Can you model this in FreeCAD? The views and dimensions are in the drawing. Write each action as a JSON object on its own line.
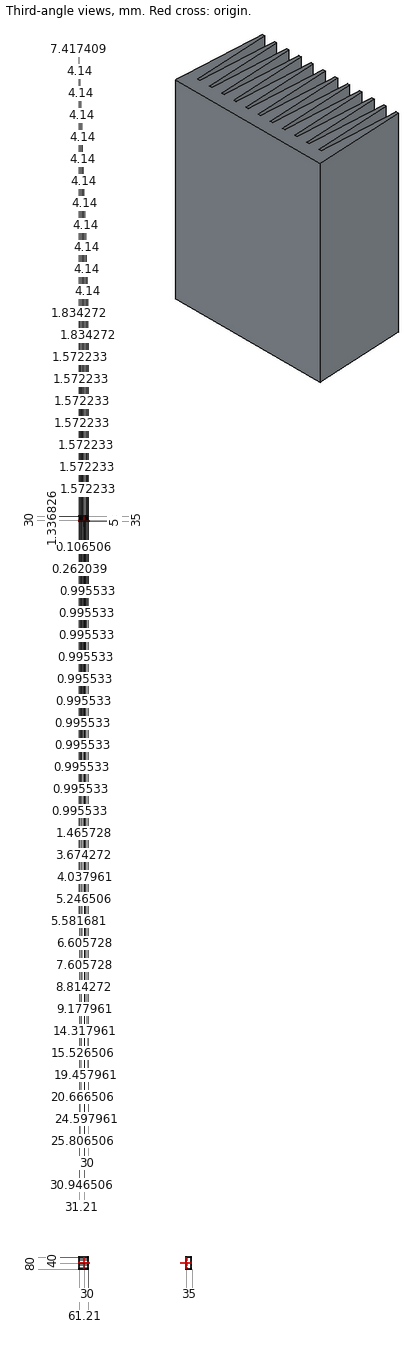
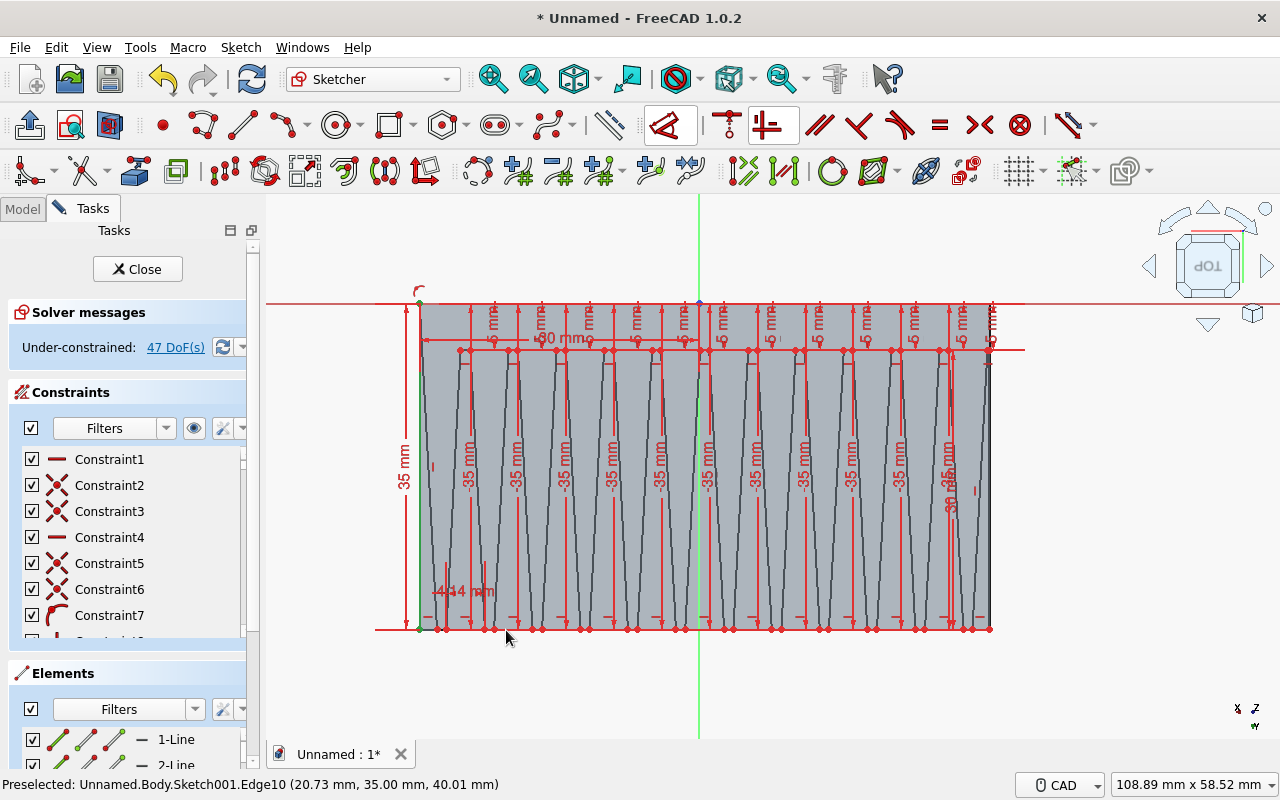
{"action": "left_click", "coordinate": [692, 126]}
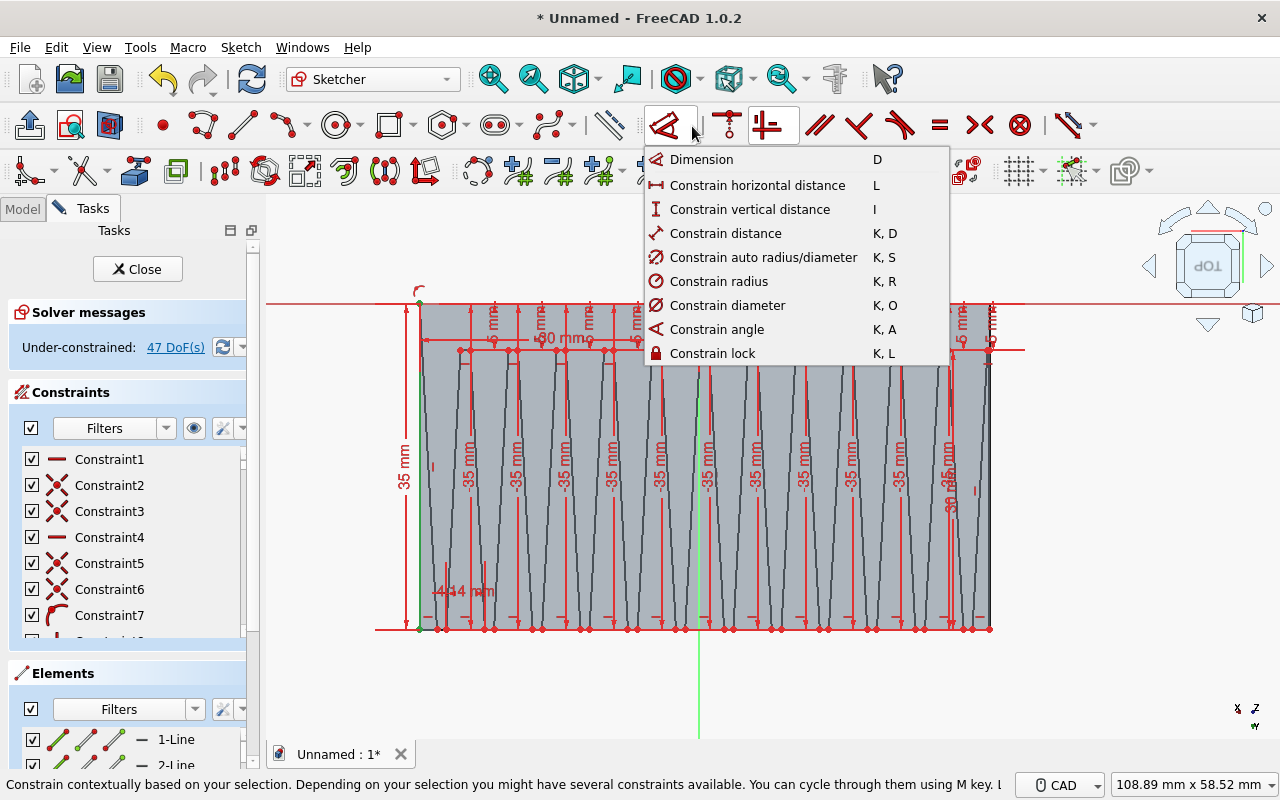
{"action": "left_click", "coordinate": [797, 185]}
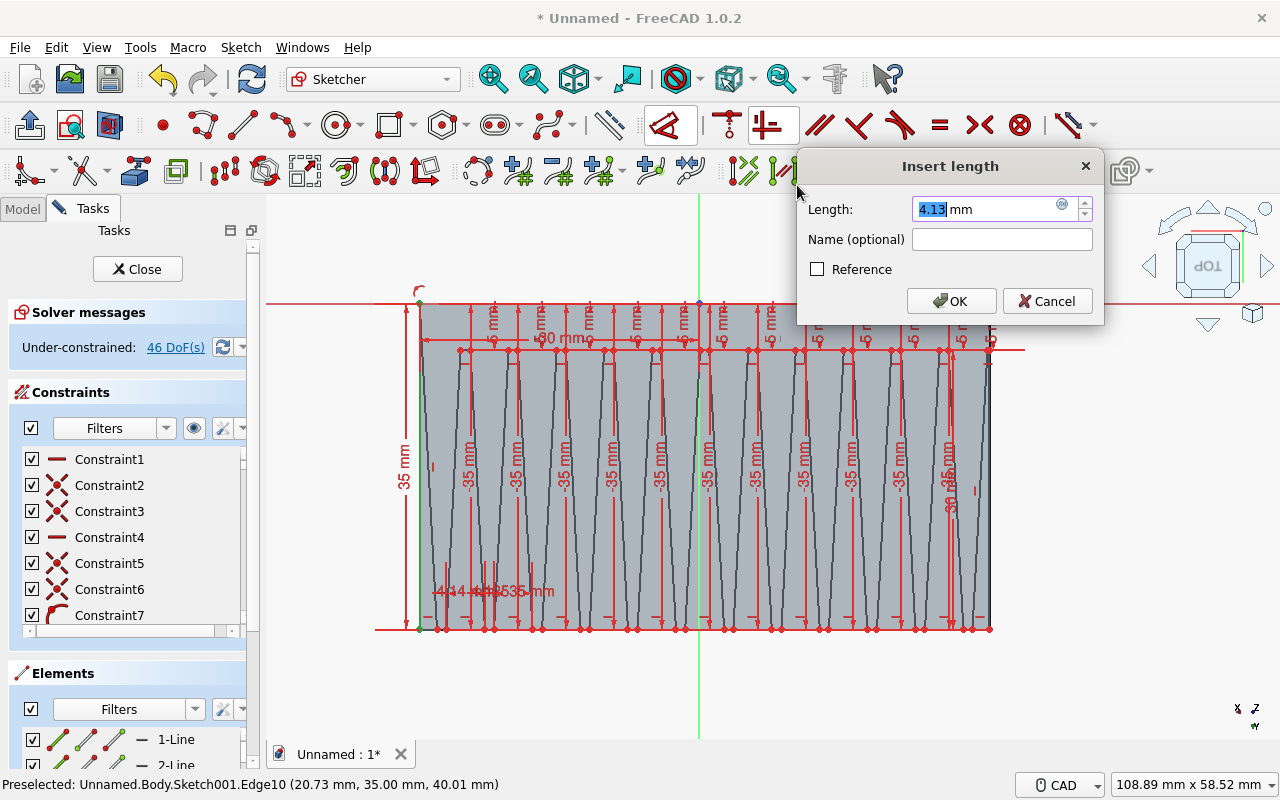
{"action": "type", "text": "4.14"}
{"action": "key", "text": "Return"}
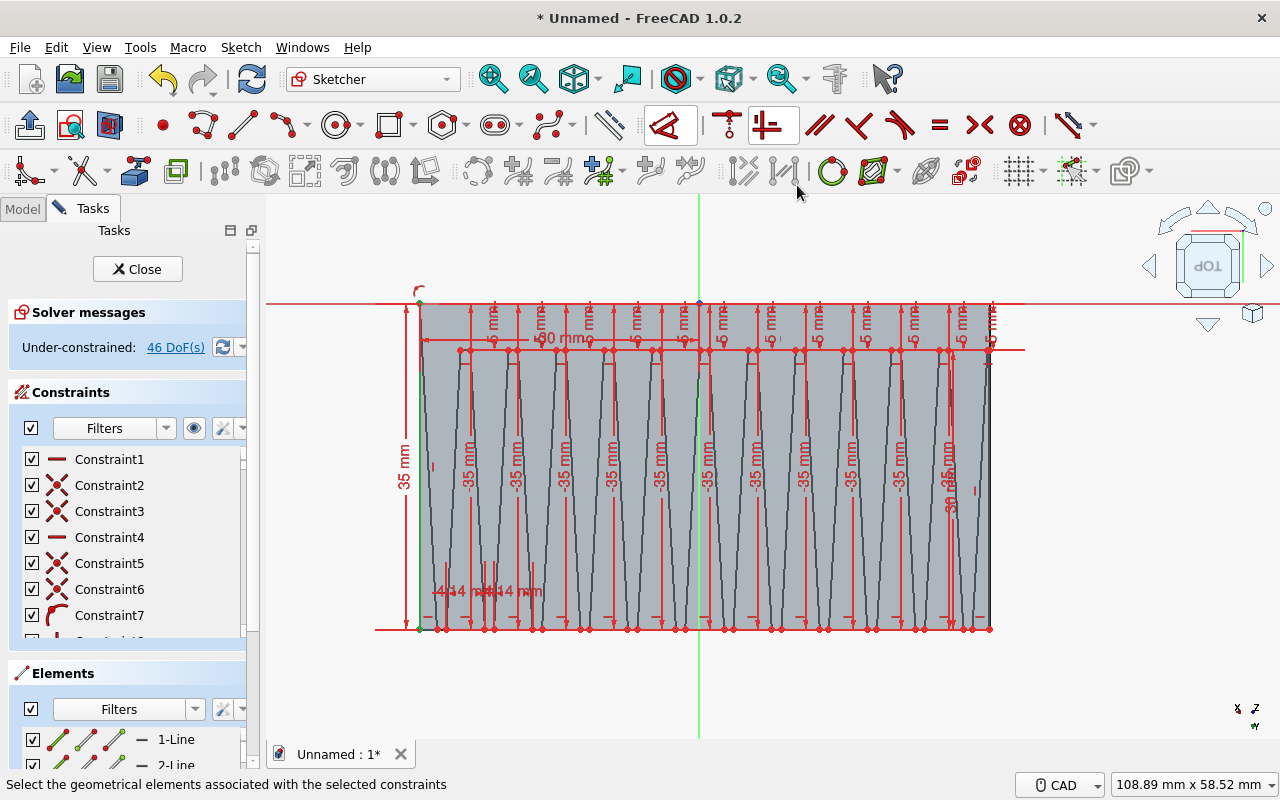
{"action": "left_click", "coordinate": [554, 630]}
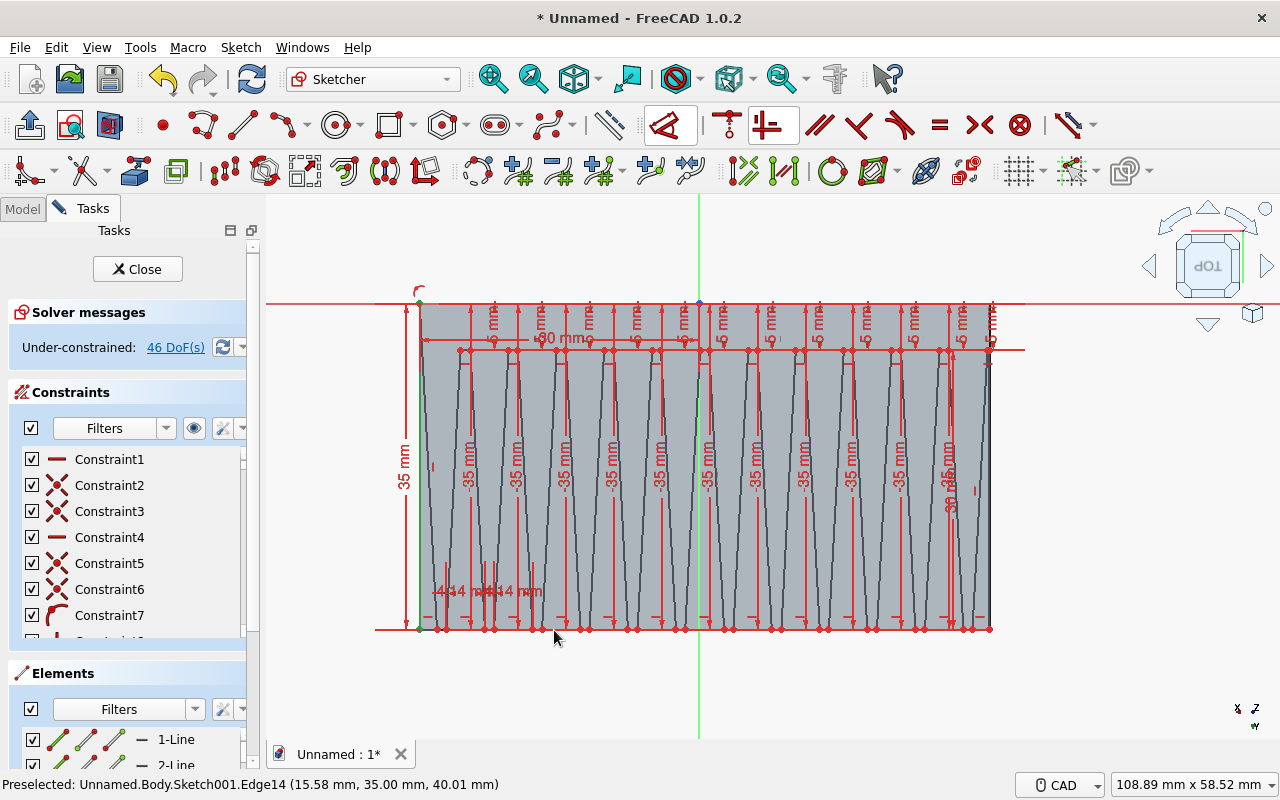
{"action": "left_click", "coordinate": [692, 126]}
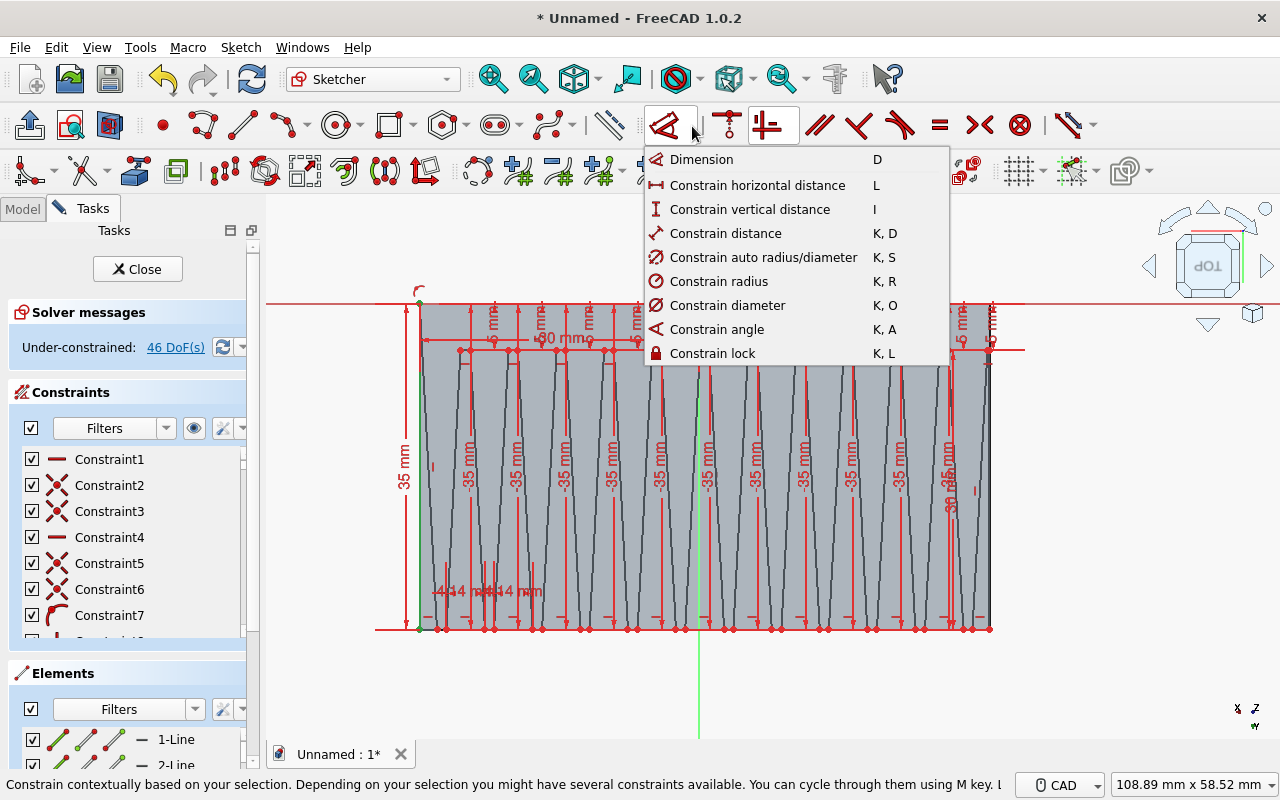
{"action": "left_click", "coordinate": [797, 185]}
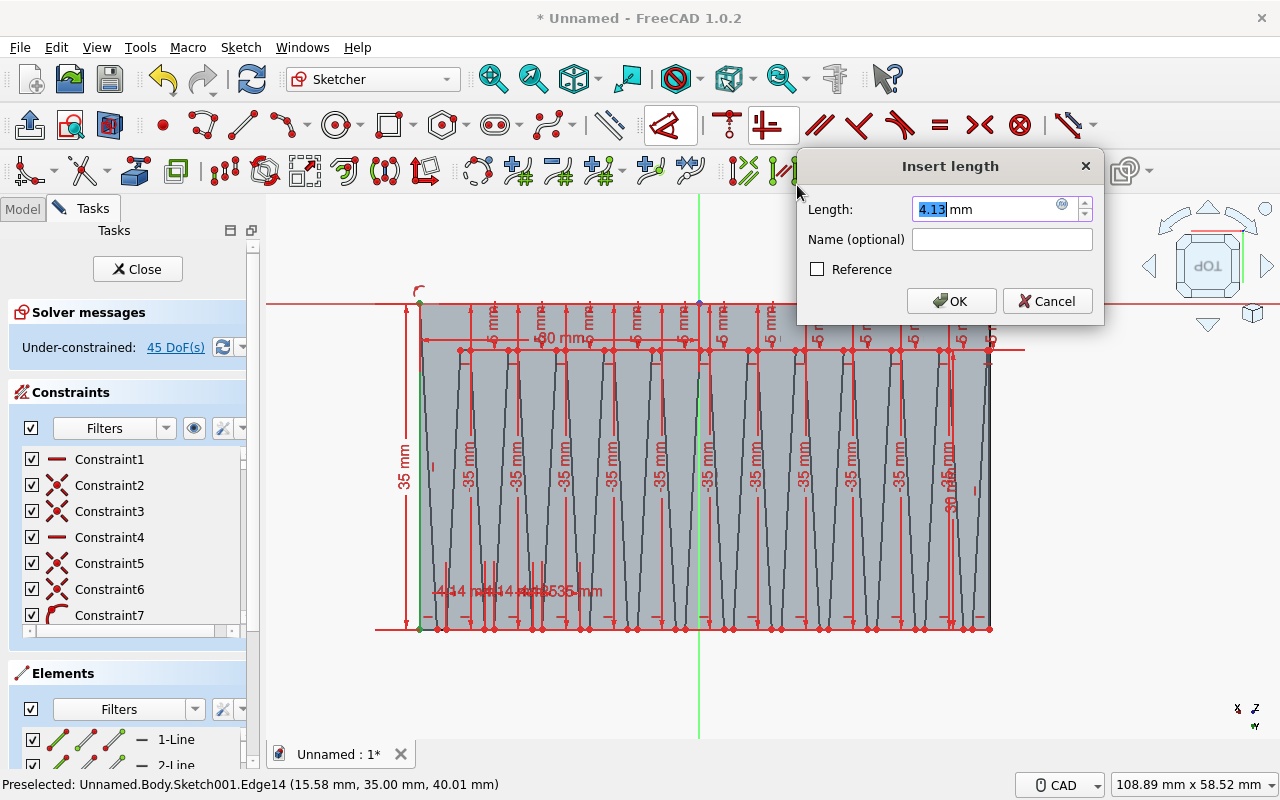
{"action": "type", "text": "4.14"}
{"action": "key", "text": "Return"}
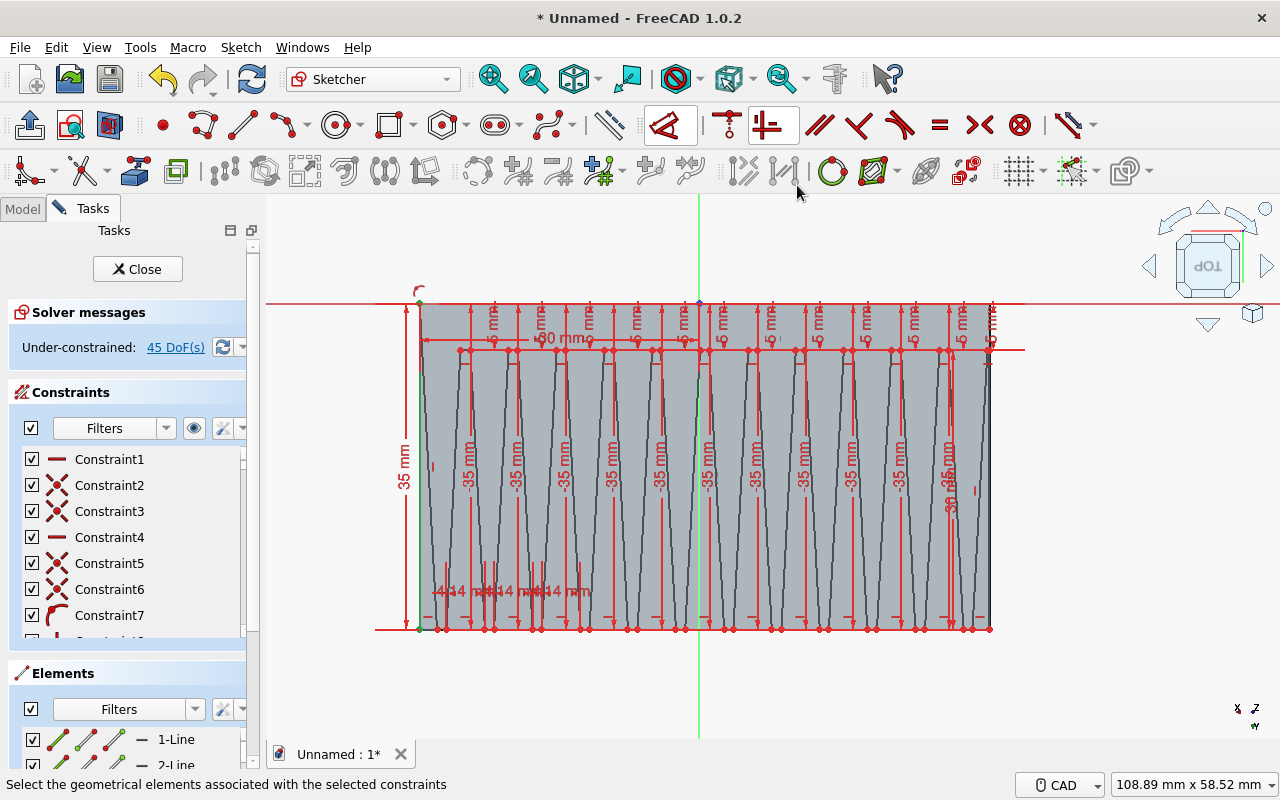
{"action": "left_click", "coordinate": [601, 630]}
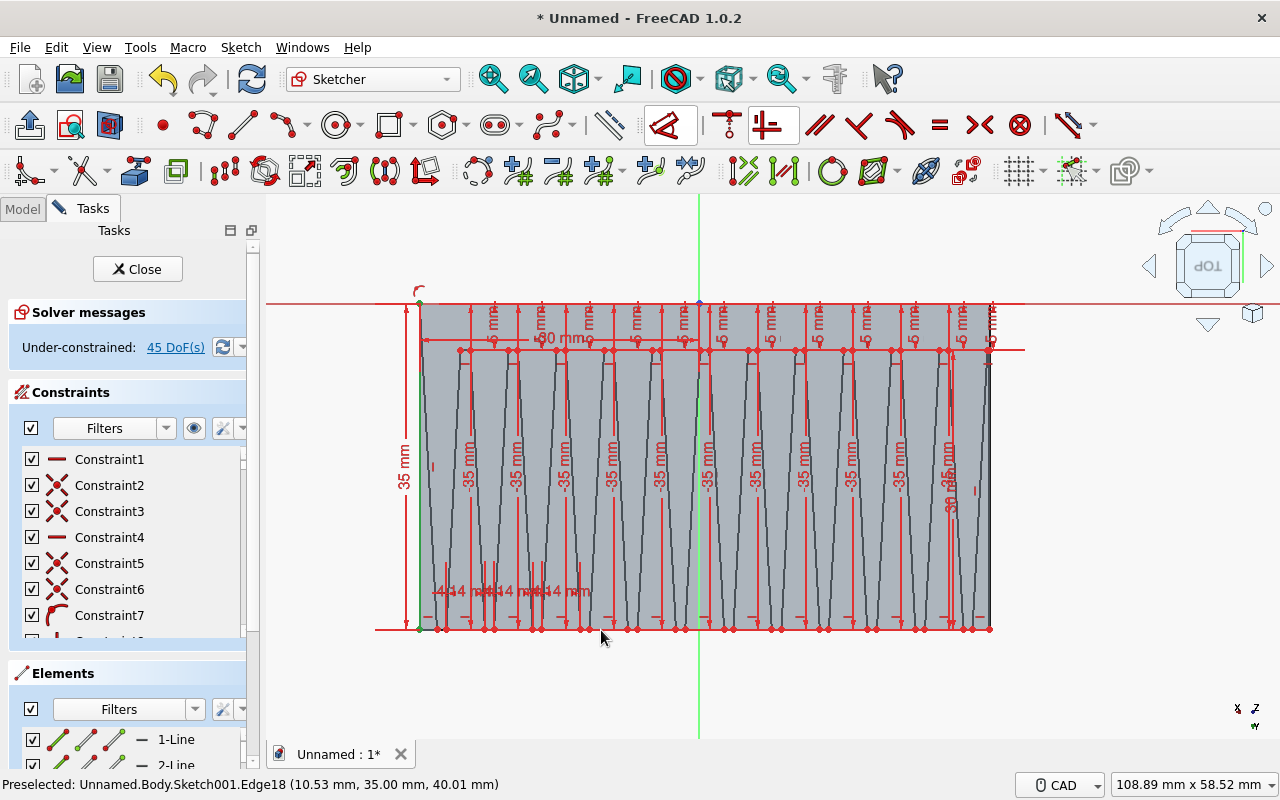
{"action": "left_click", "coordinate": [692, 126]}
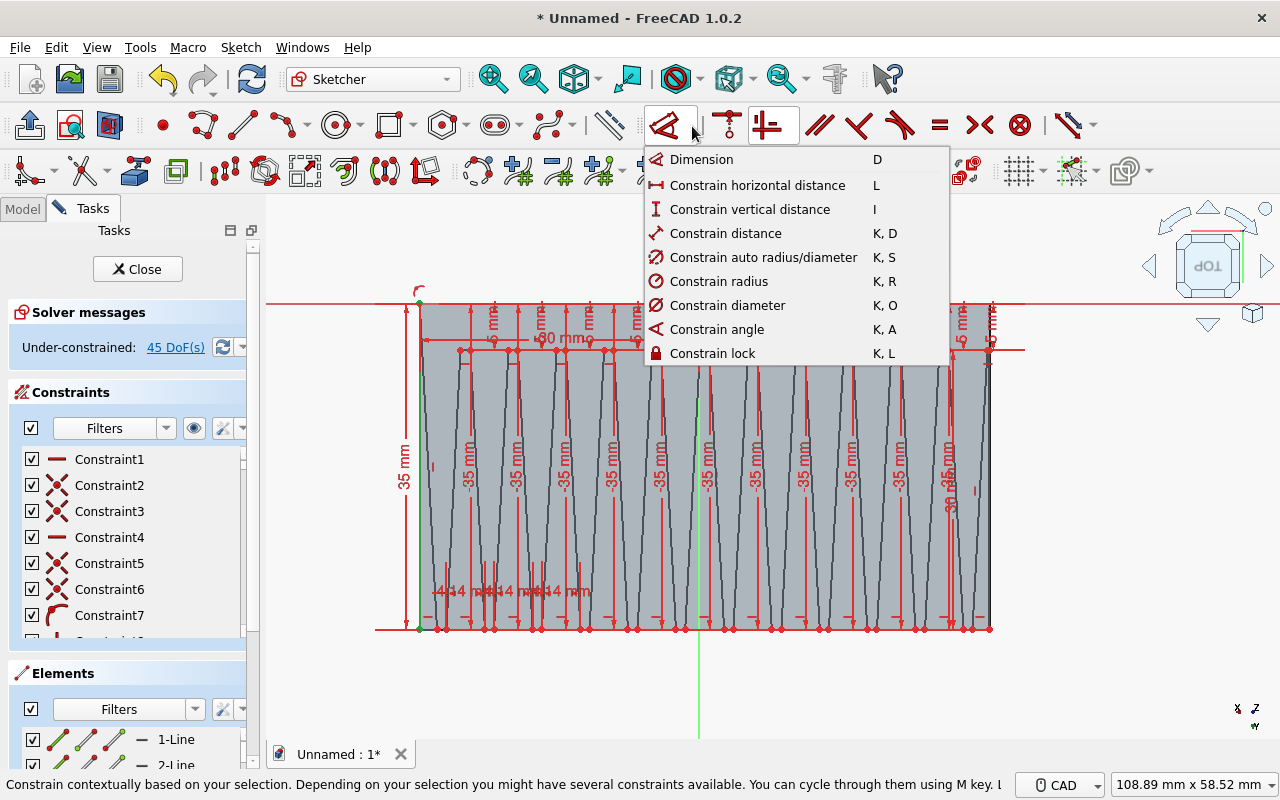
{"action": "left_click", "coordinate": [797, 185]}